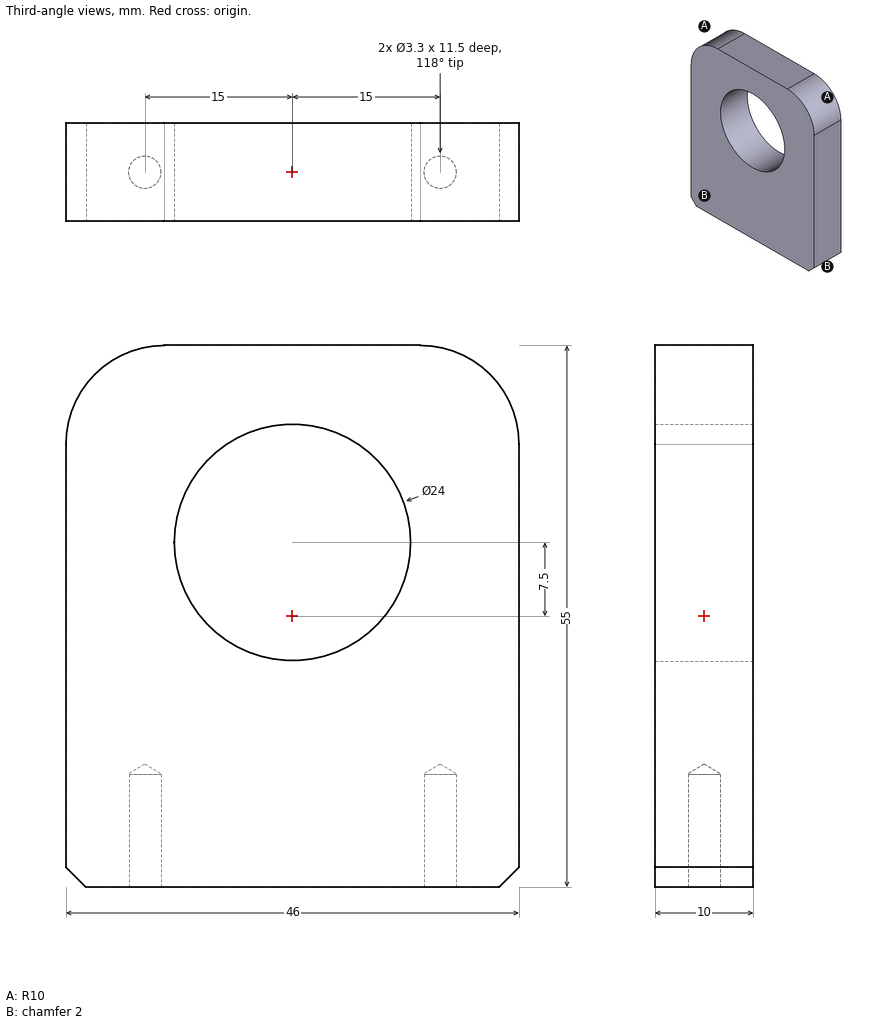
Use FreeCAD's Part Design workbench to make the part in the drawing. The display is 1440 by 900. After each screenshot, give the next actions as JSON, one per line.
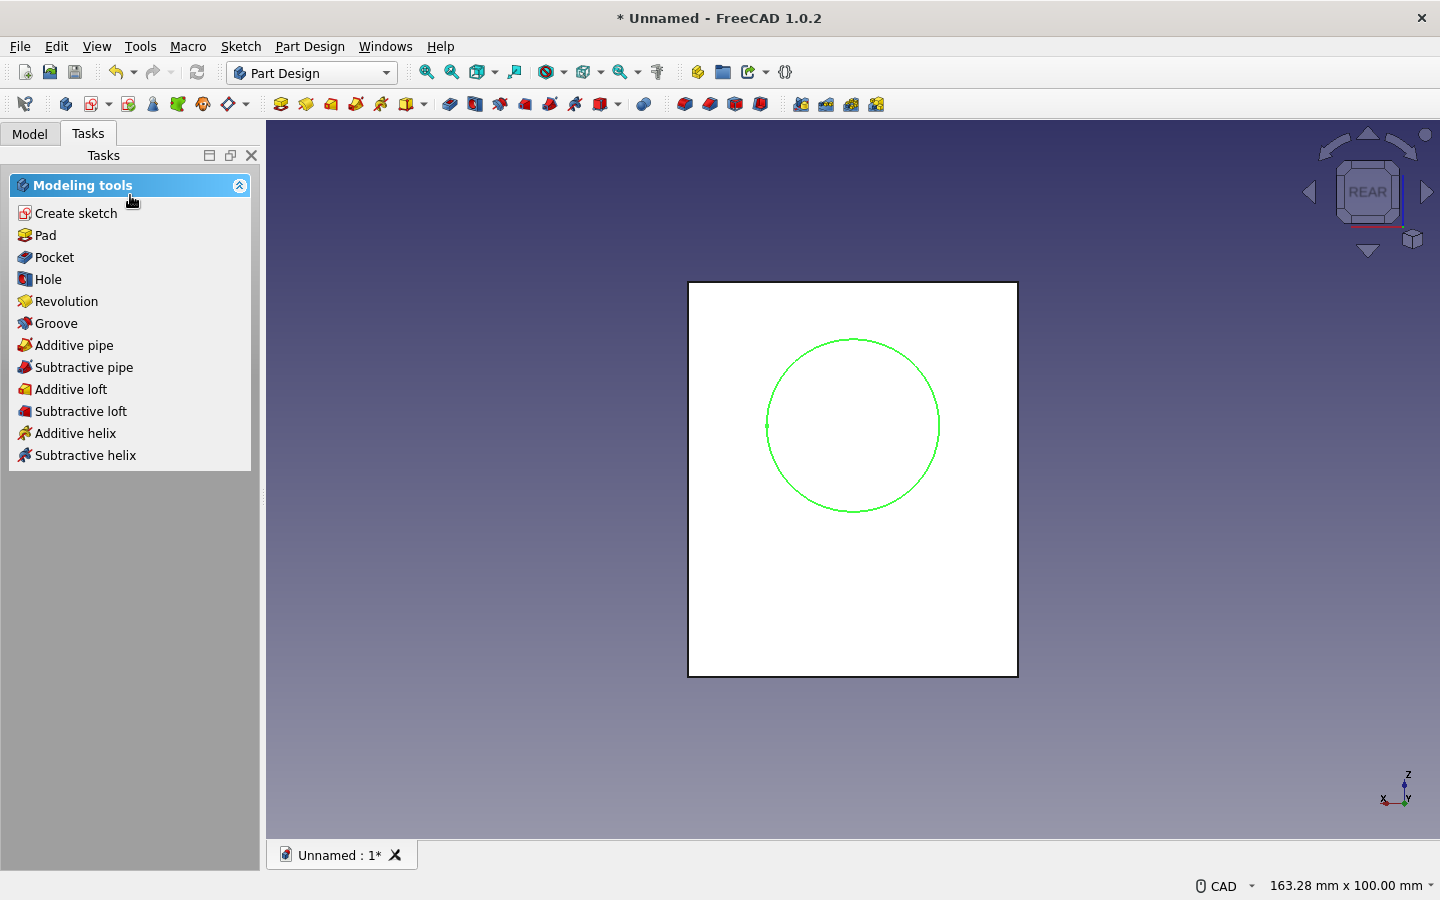
{"action": "left_click", "coordinate": [450, 104]}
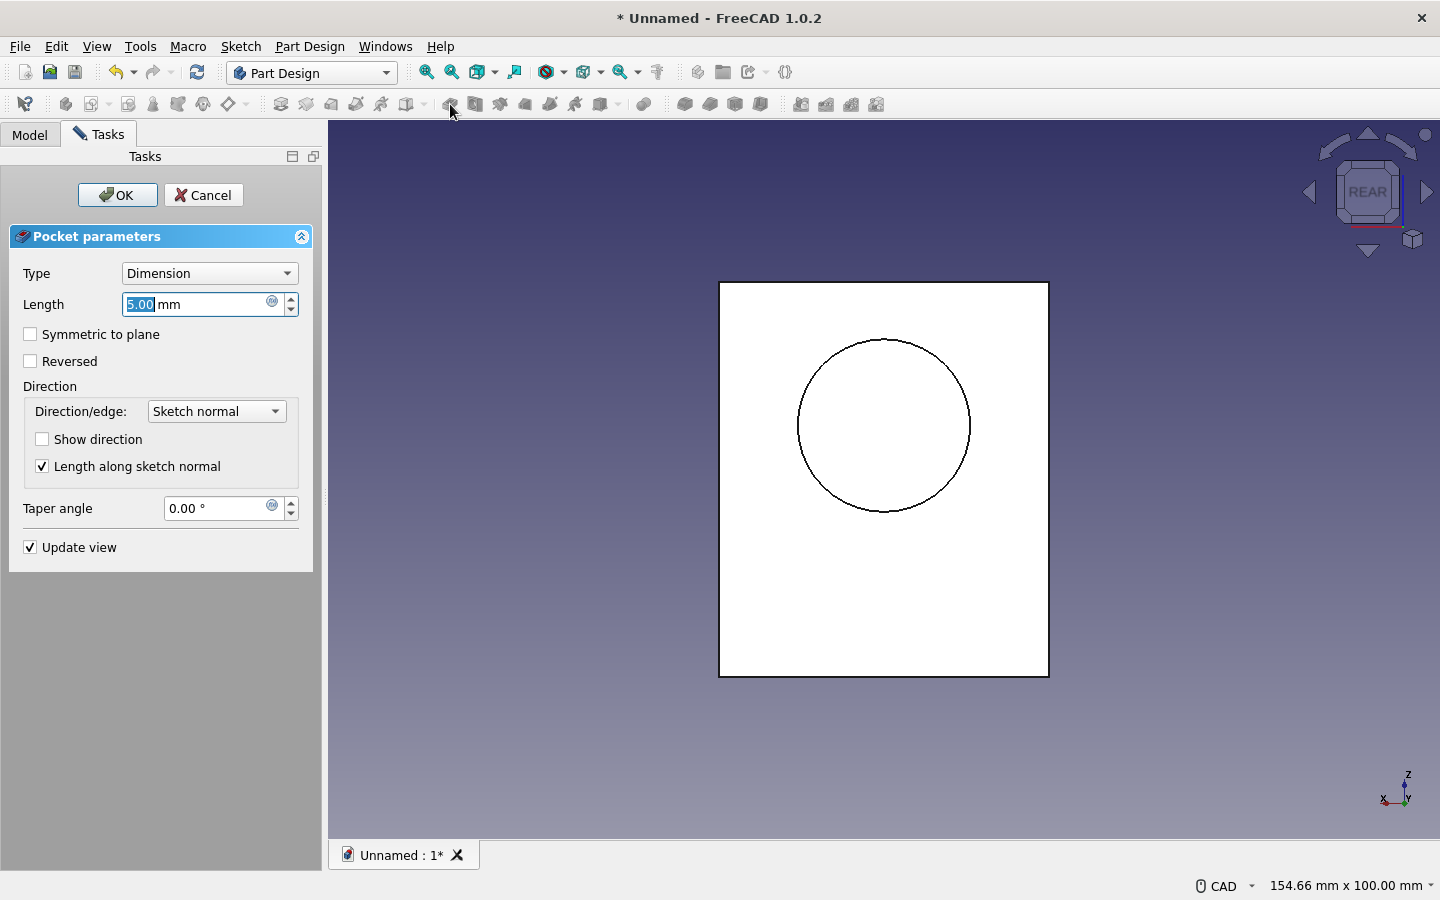
{"action": "left_click", "coordinate": [210, 274]}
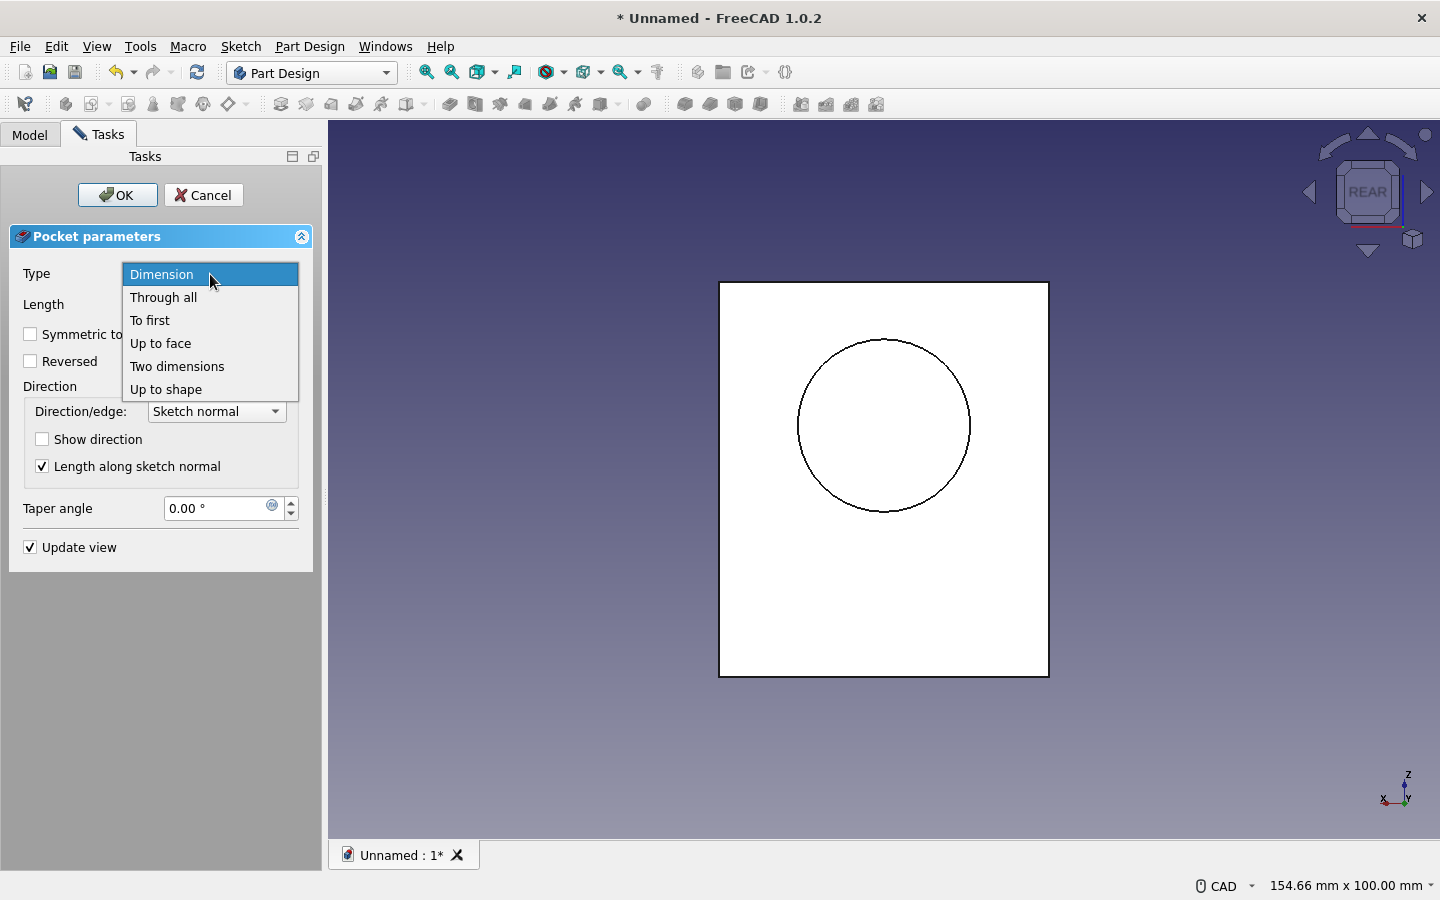
{"action": "left_click", "coordinate": [208, 298]}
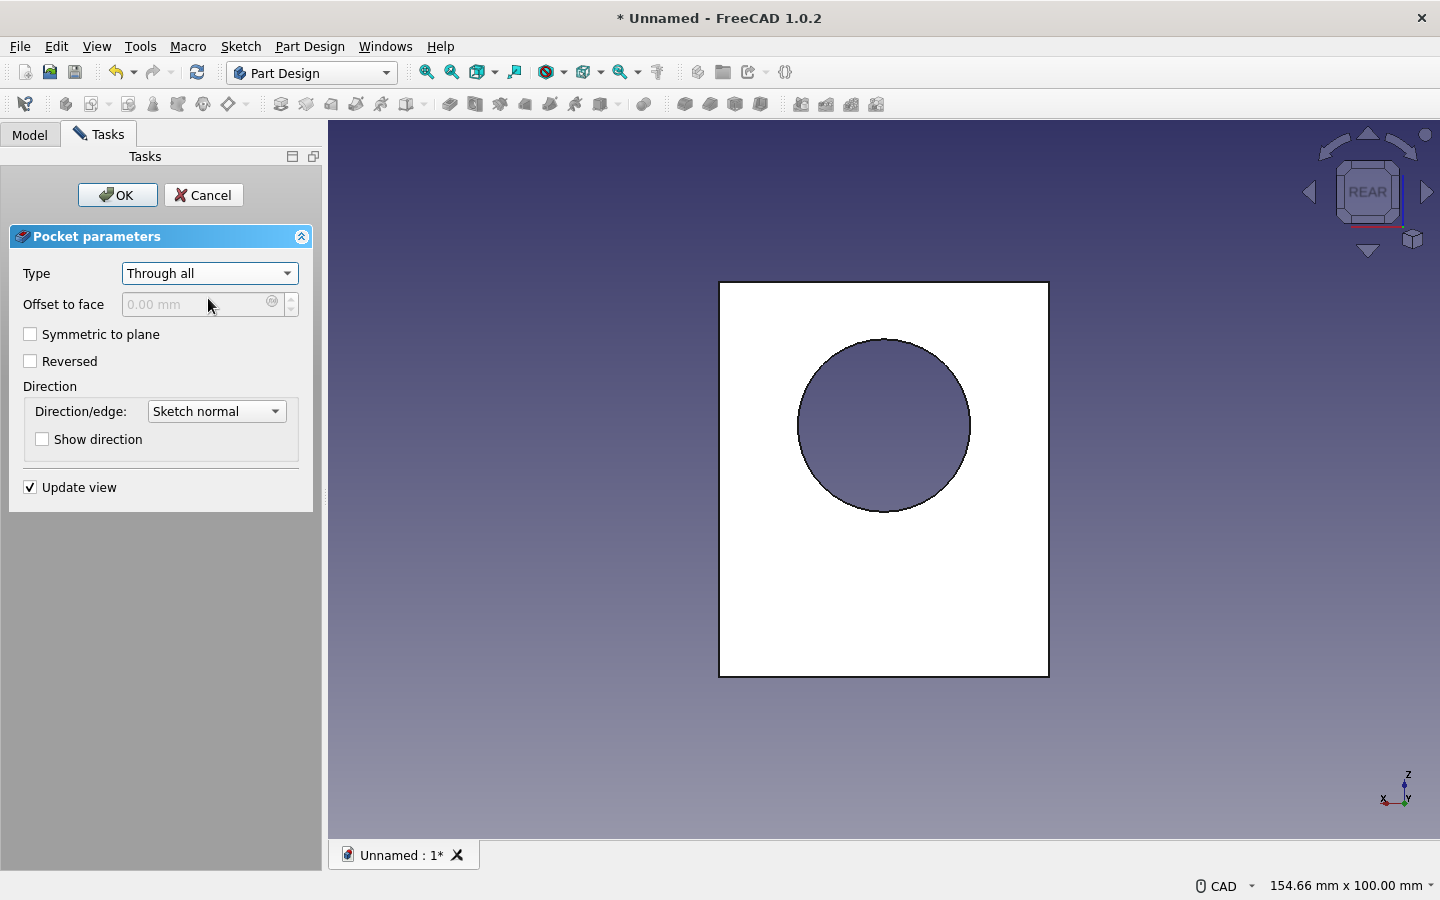
{"action": "left_click", "coordinate": [118, 195]}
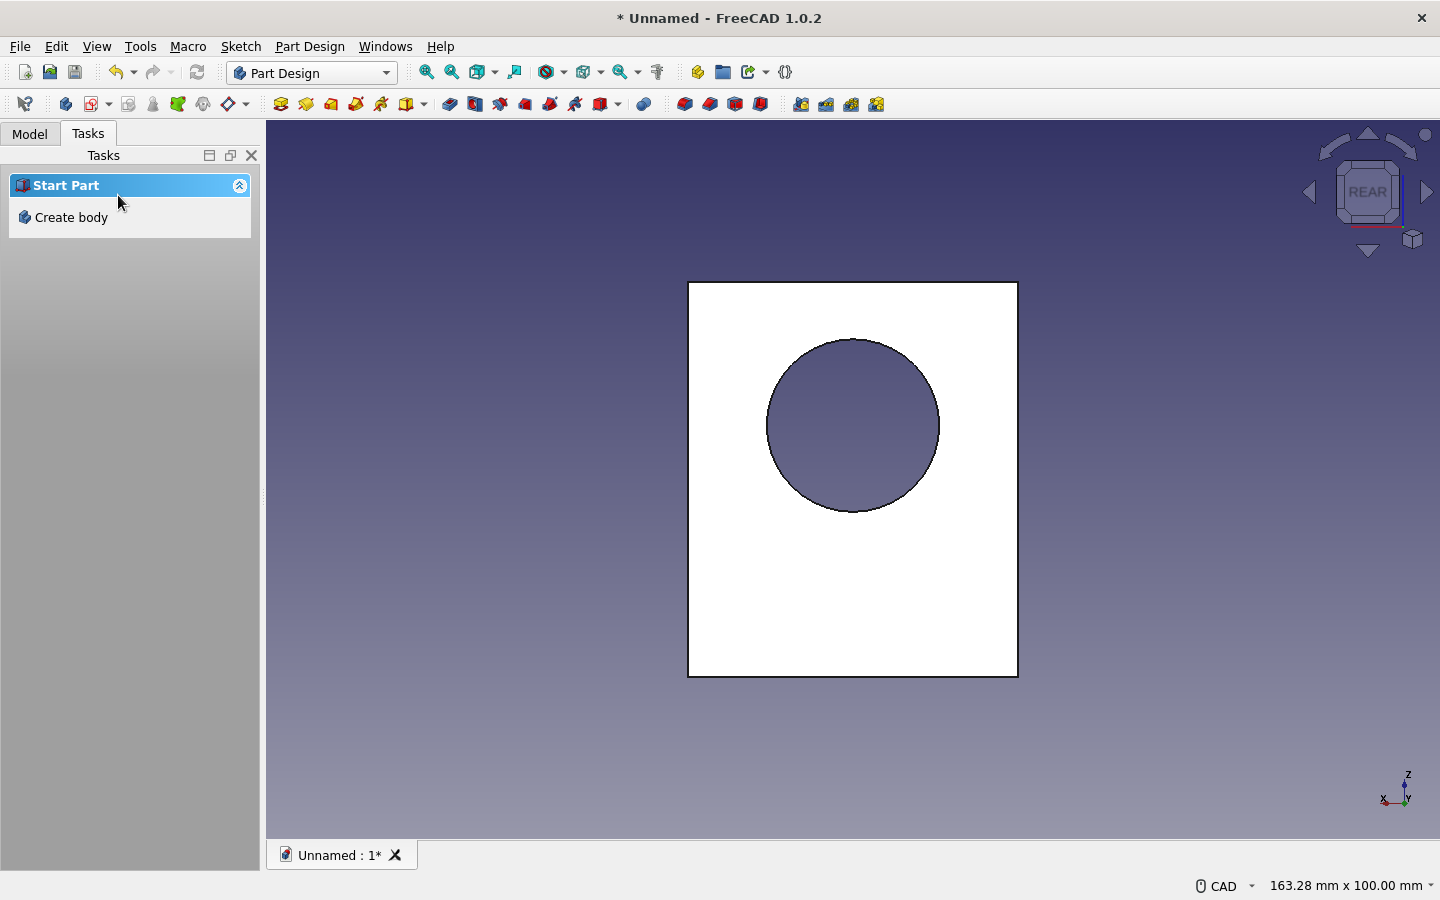
{"action": "key", "text": "0"}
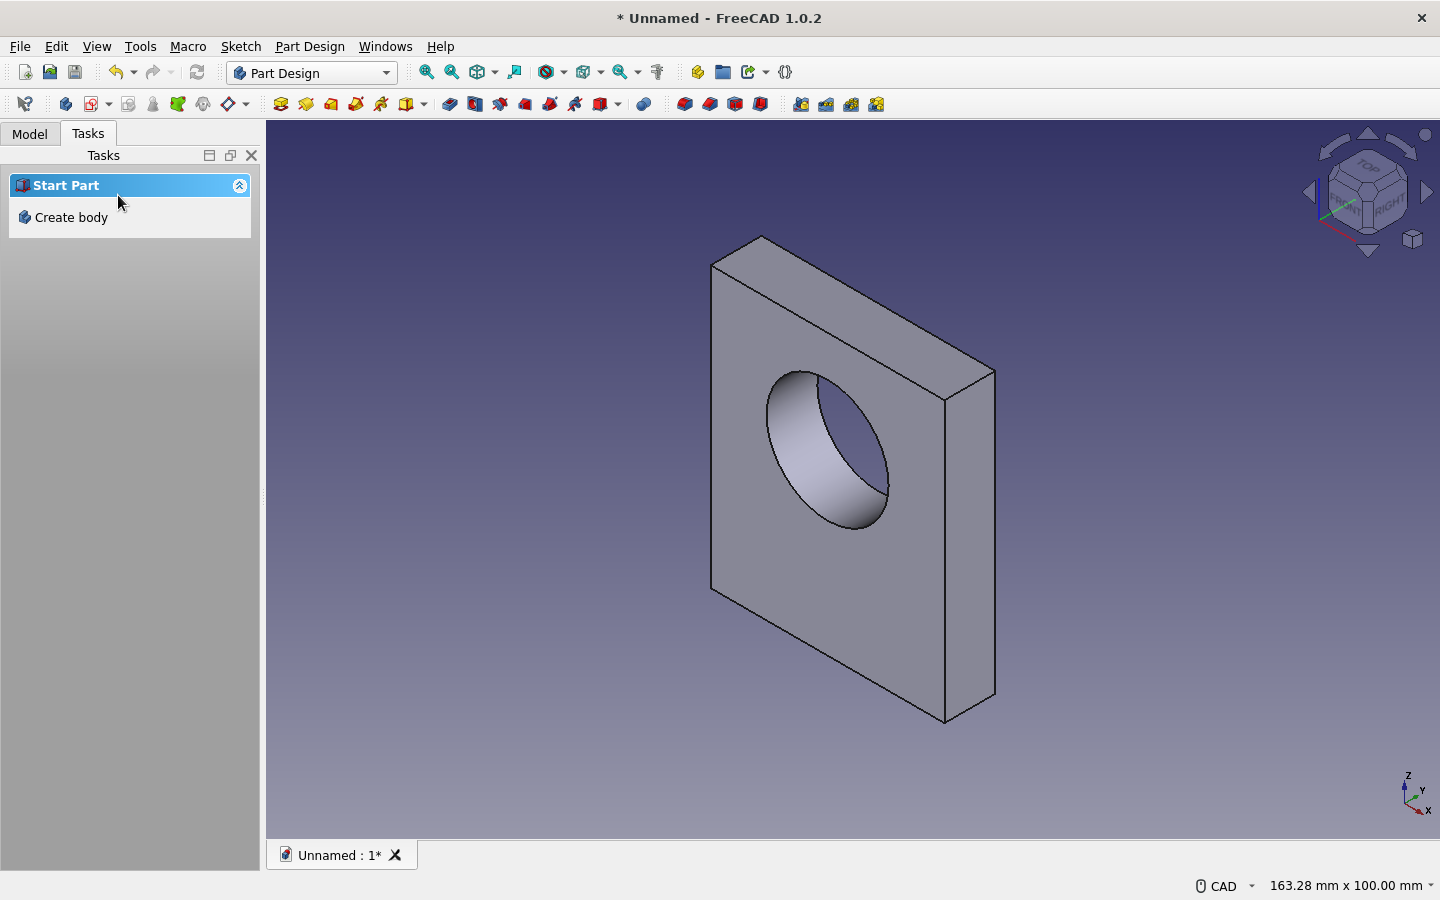
{"action": "left_click", "coordinate": [970, 385]}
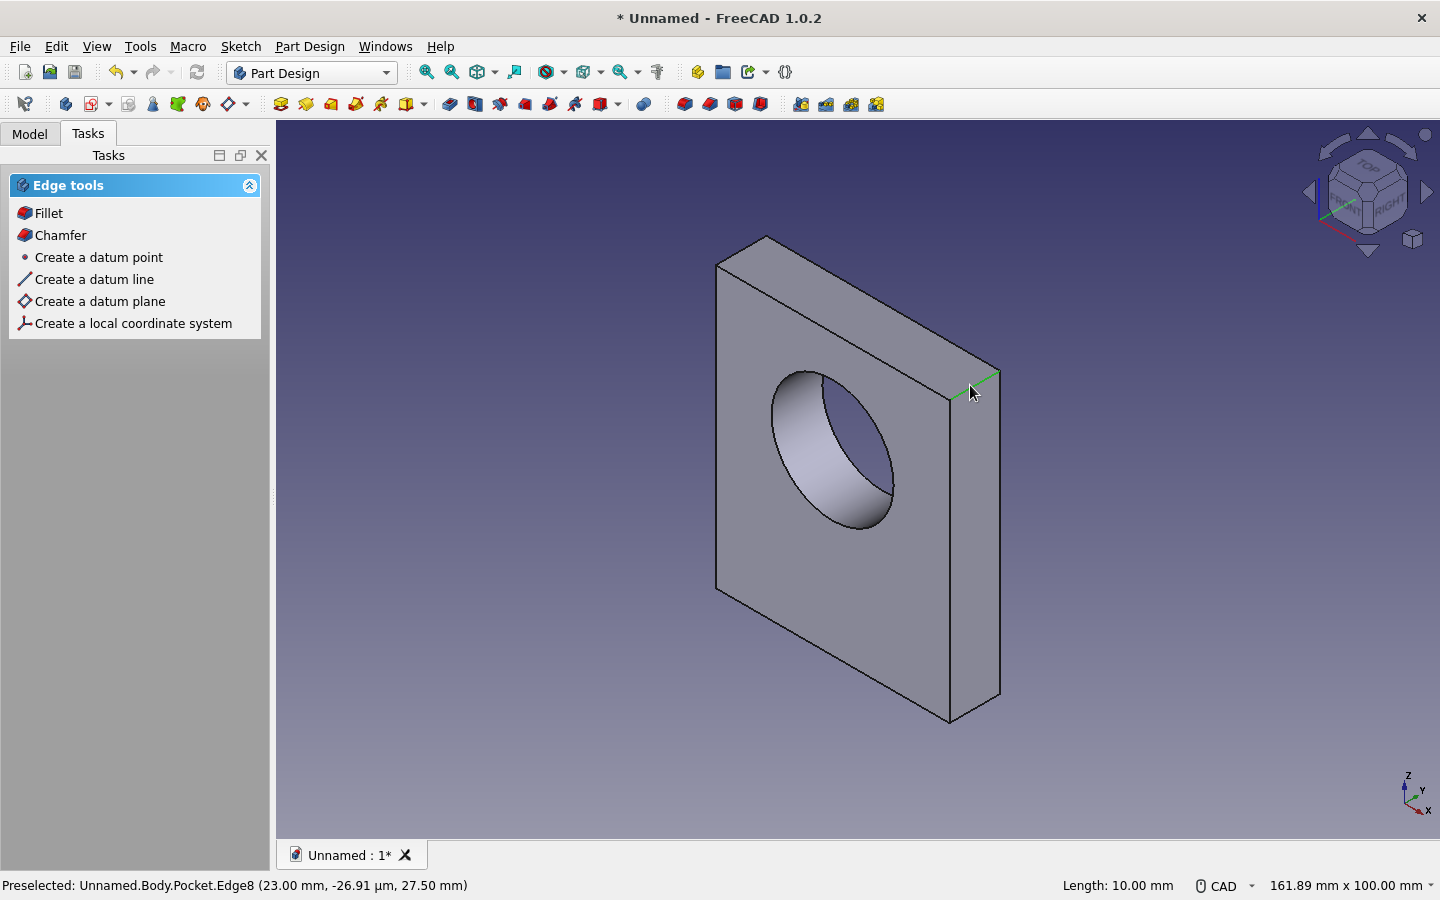
{"action": "key", "text": "2"}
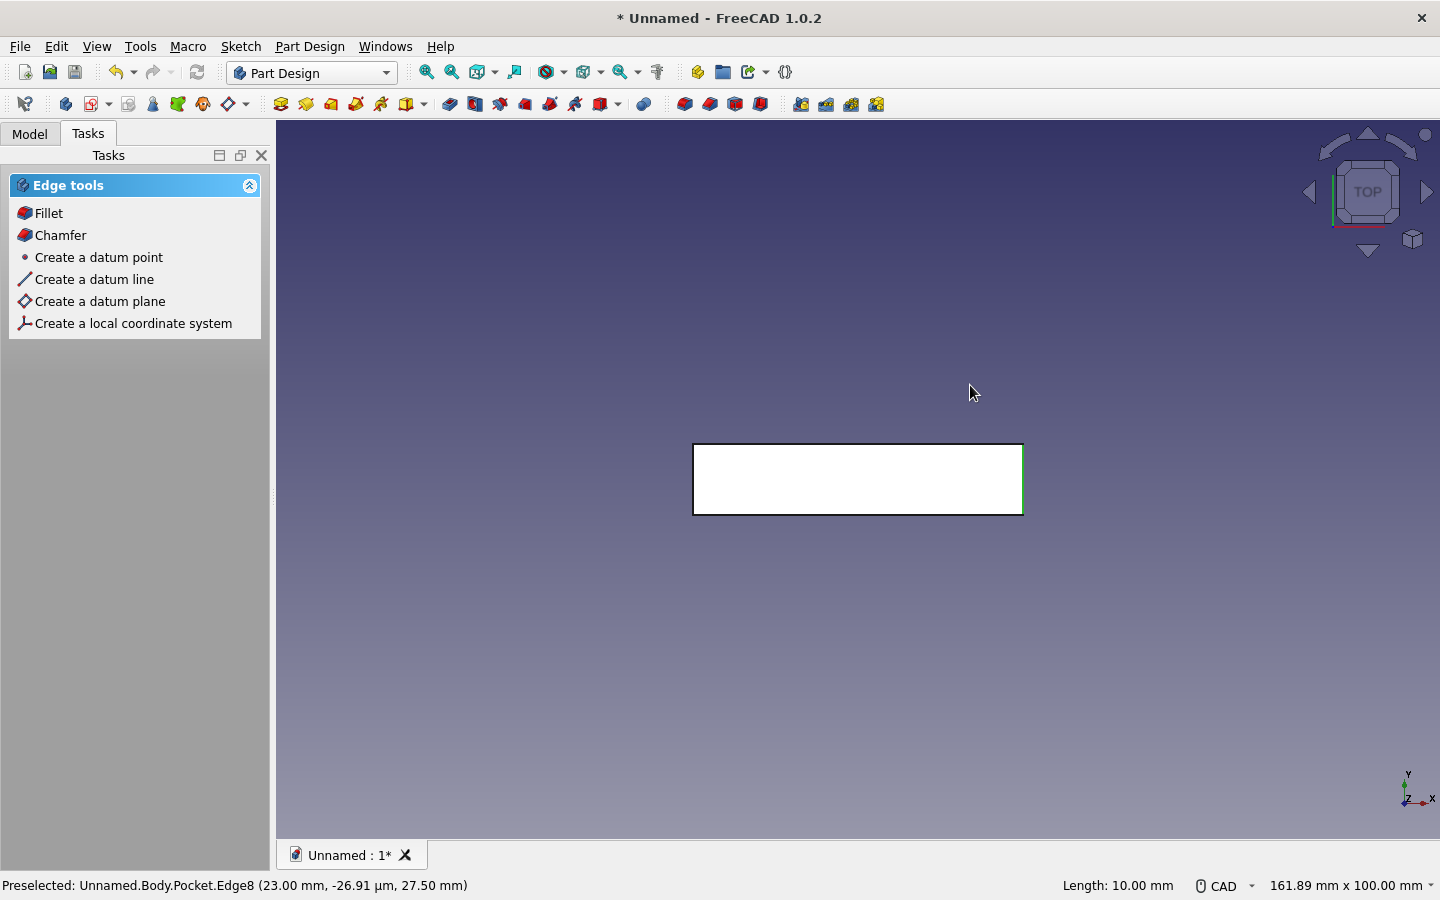
{"action": "left_click", "coordinate": [427, 72]}